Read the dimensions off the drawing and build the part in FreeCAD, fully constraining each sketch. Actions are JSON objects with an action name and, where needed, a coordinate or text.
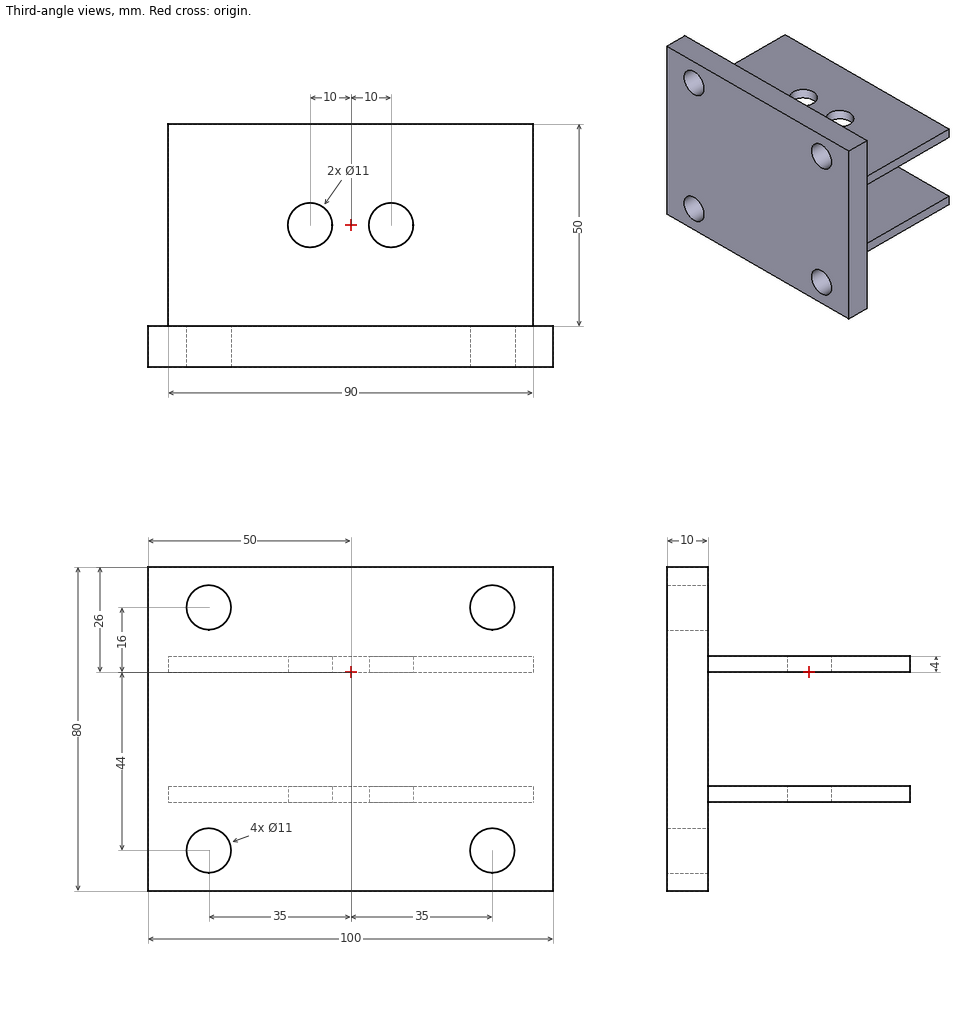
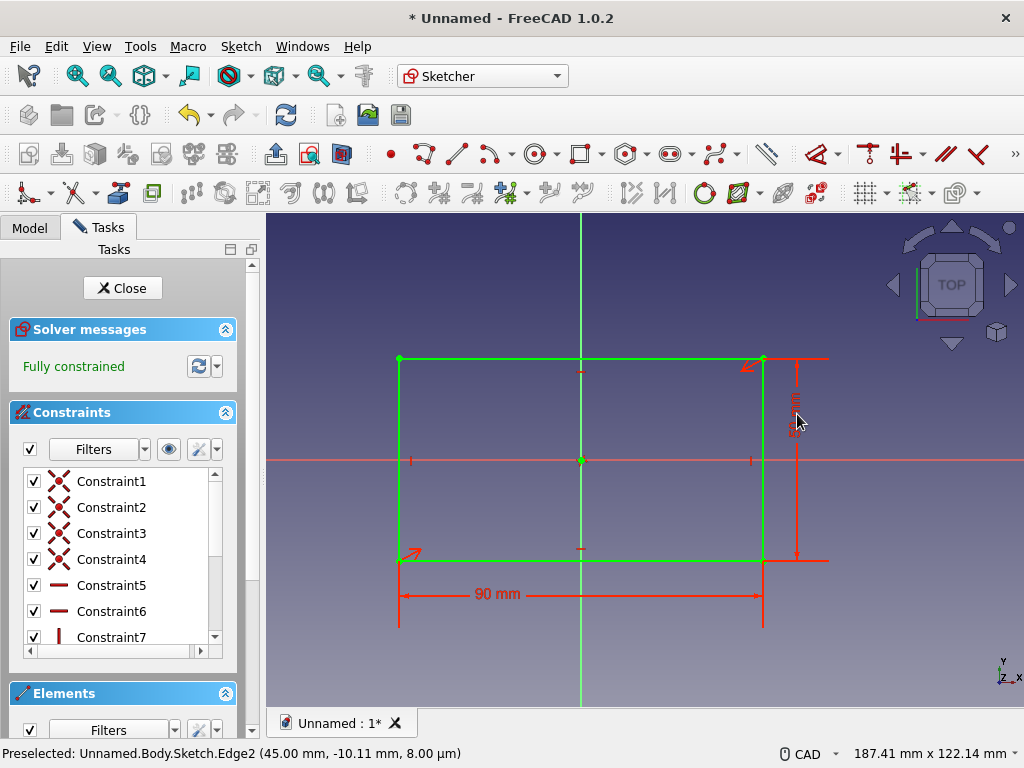
{"action": "left_click", "coordinate": [123, 288]}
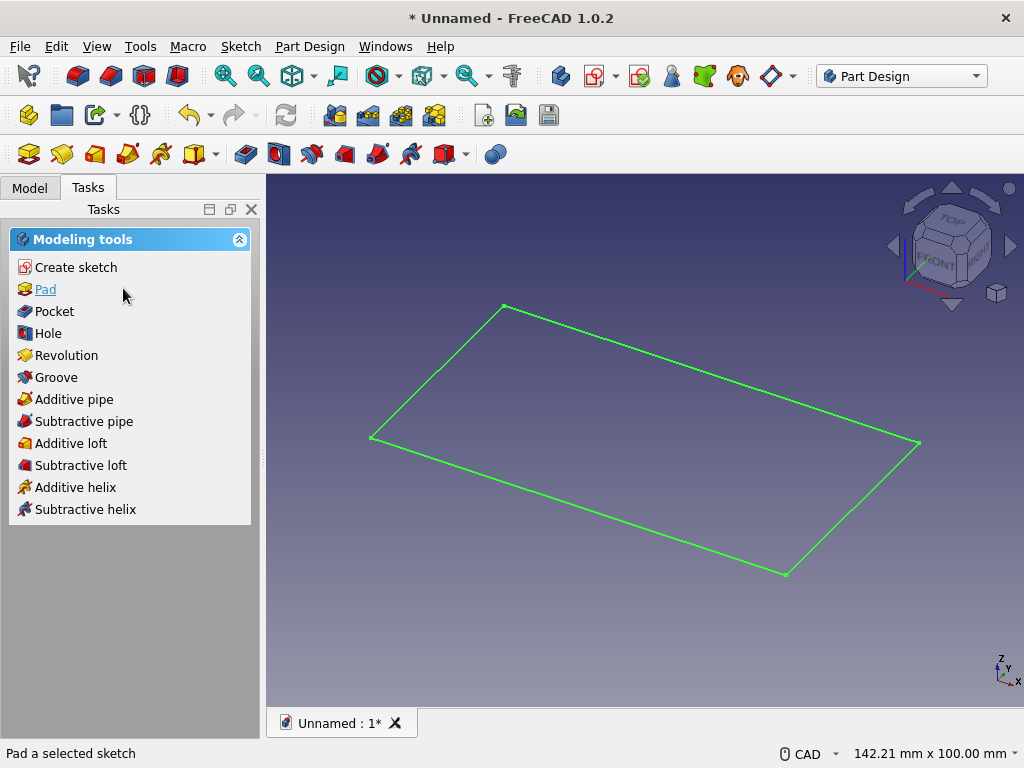
{"action": "left_click", "coordinate": [29, 154]}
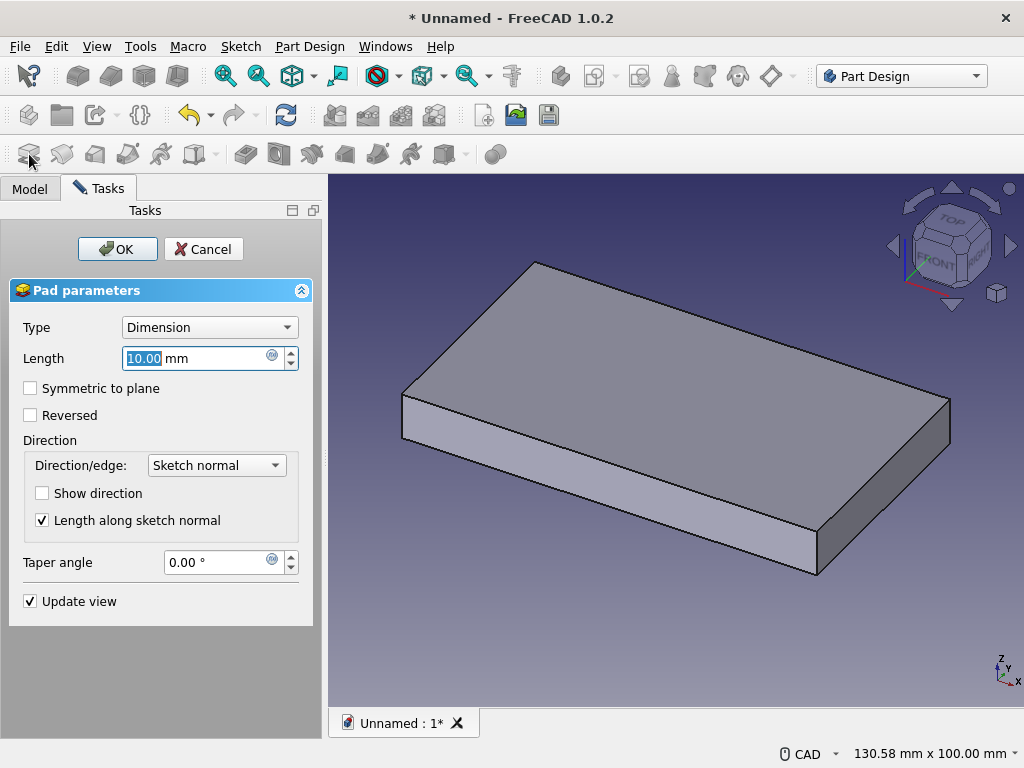
{"action": "type", "text": "4"}
{"action": "key", "text": "Tab"}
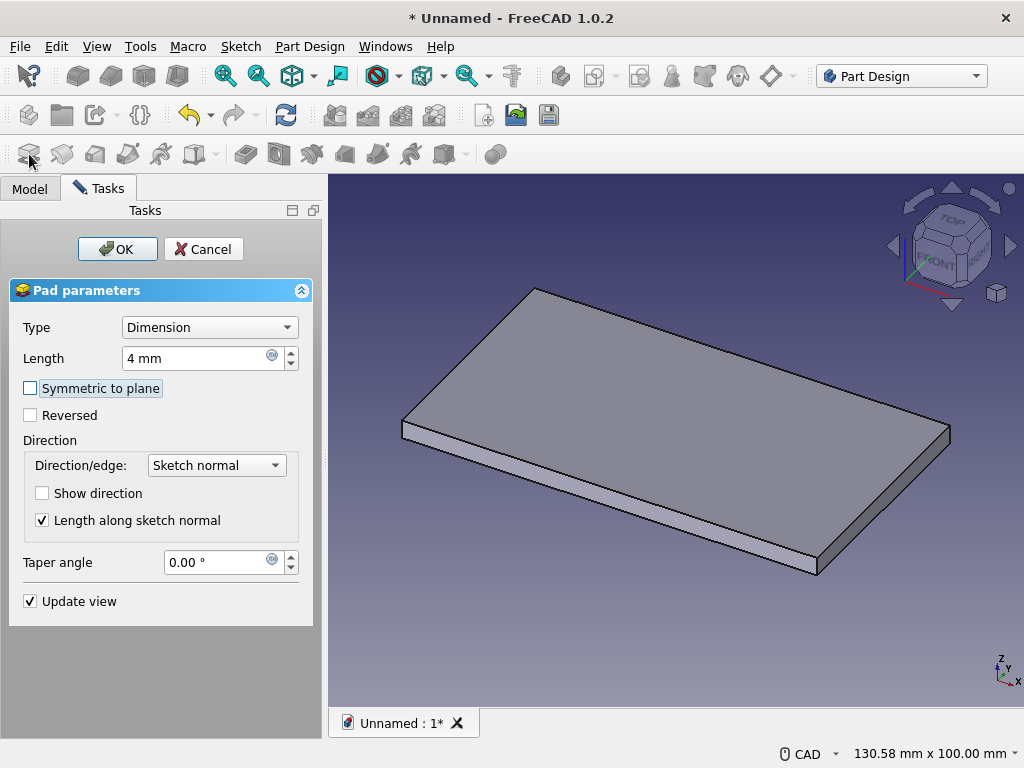
{"action": "left_click", "coordinate": [118, 249]}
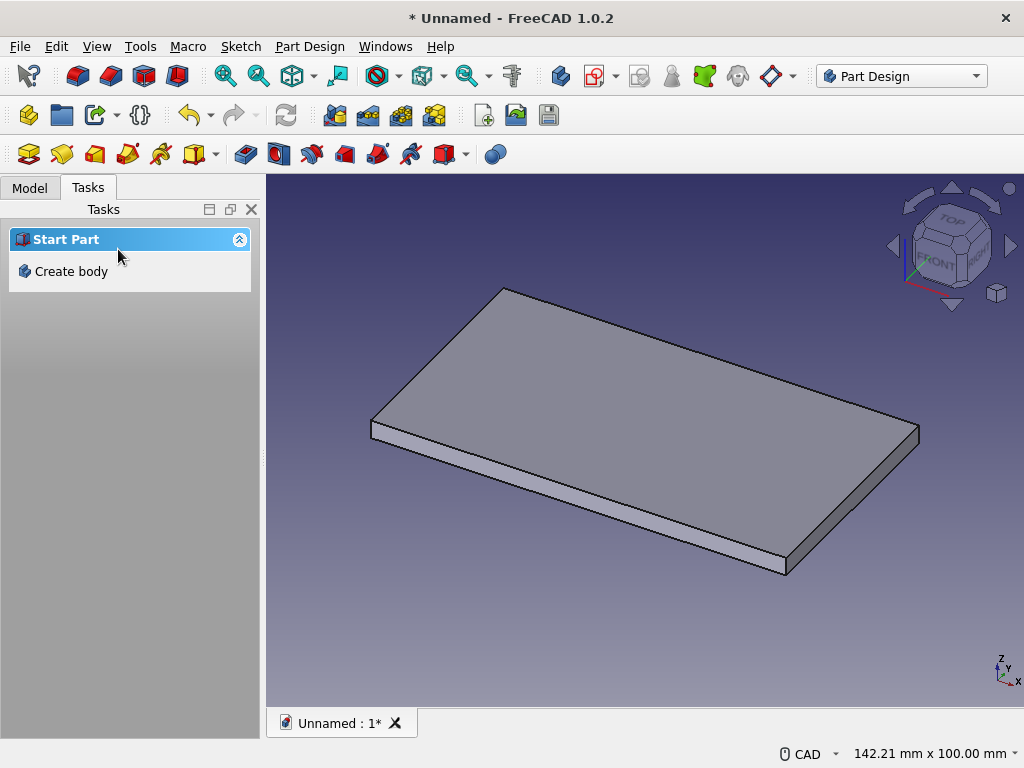
{"action": "left_click", "coordinate": [704, 442]}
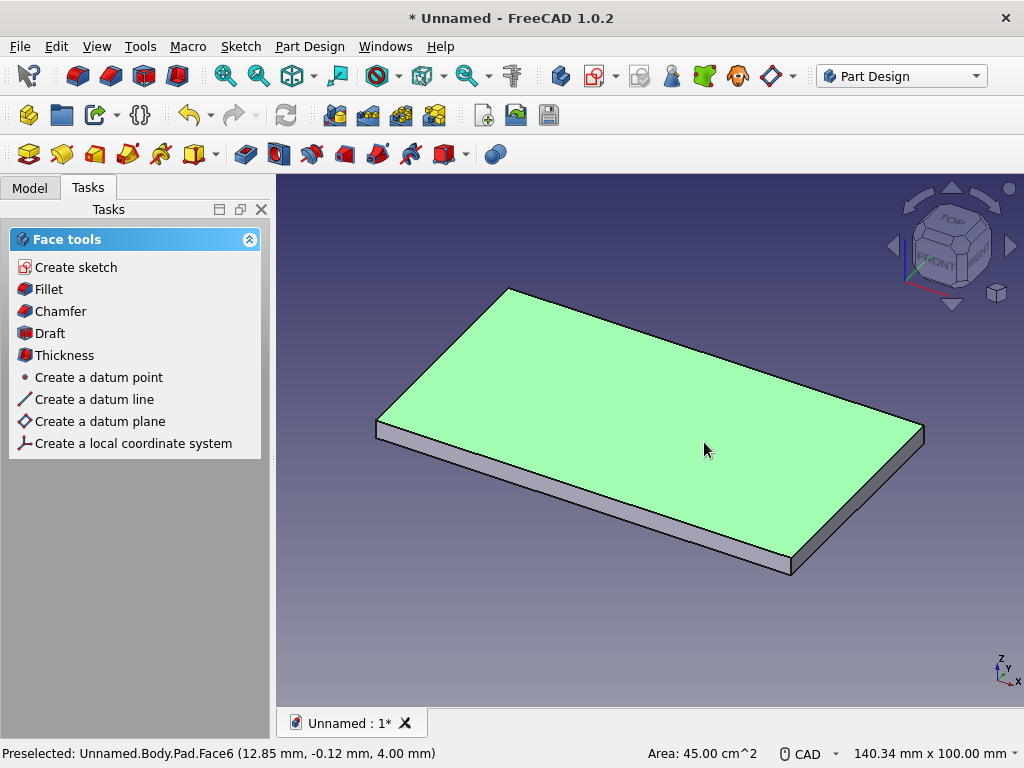
{"action": "left_click", "coordinate": [594, 76]}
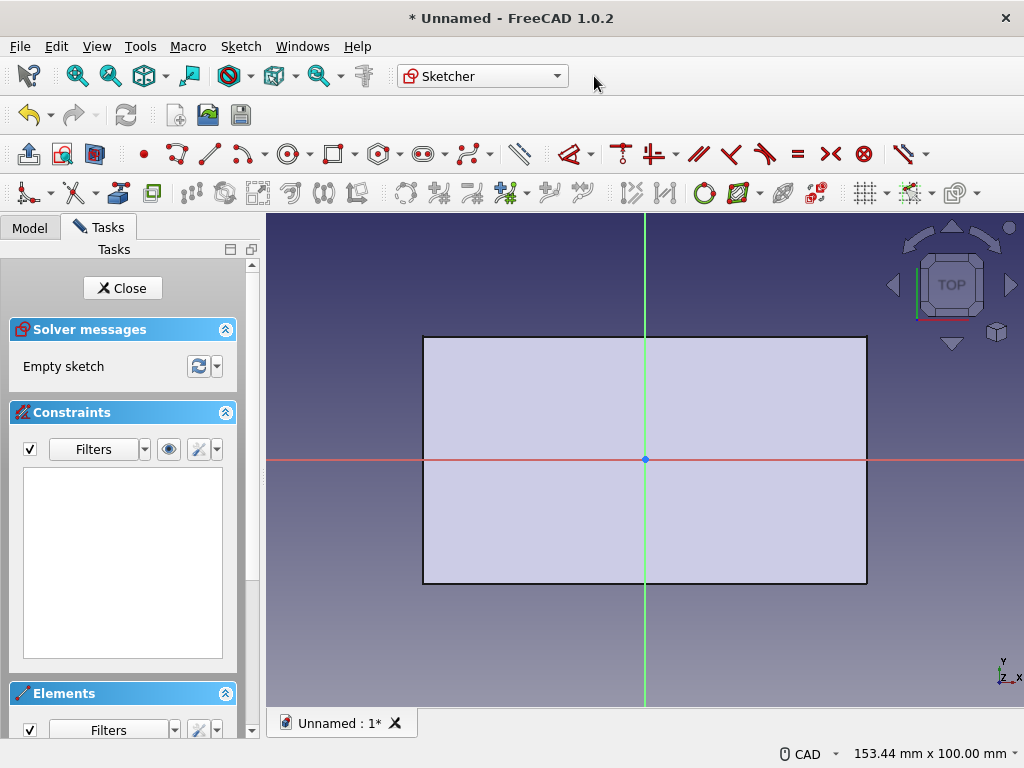
{"action": "scroll", "coordinate": [685, 460], "scroll_direction": "up", "scroll_amount": 5}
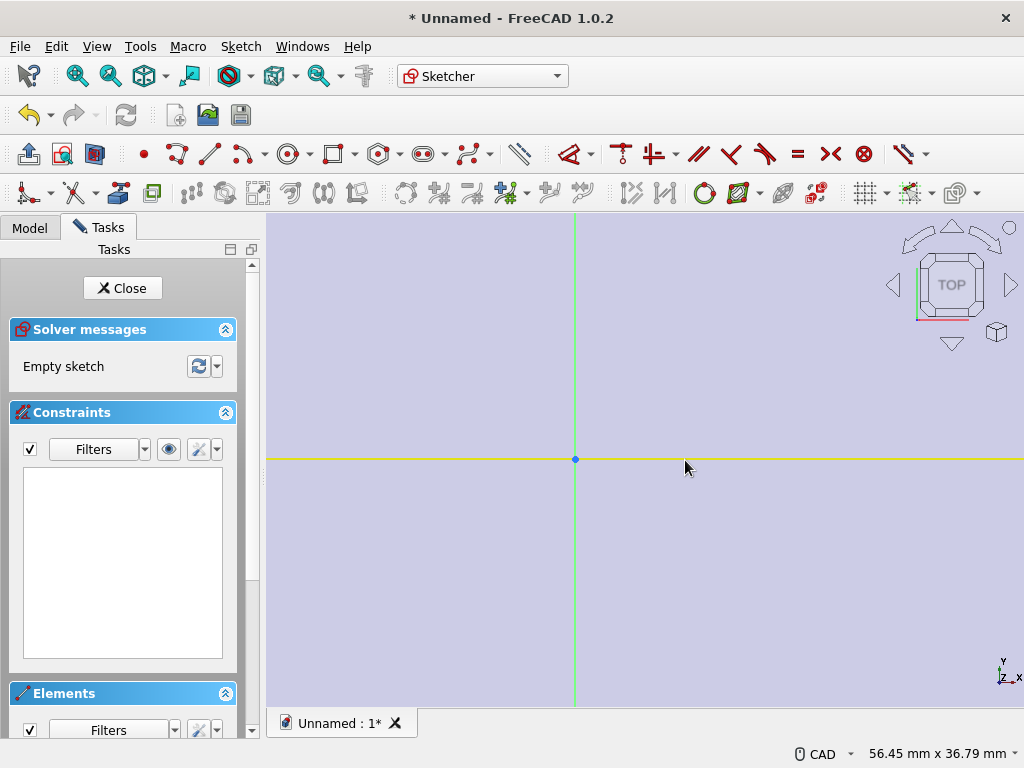
{"action": "key", "text": "g c"}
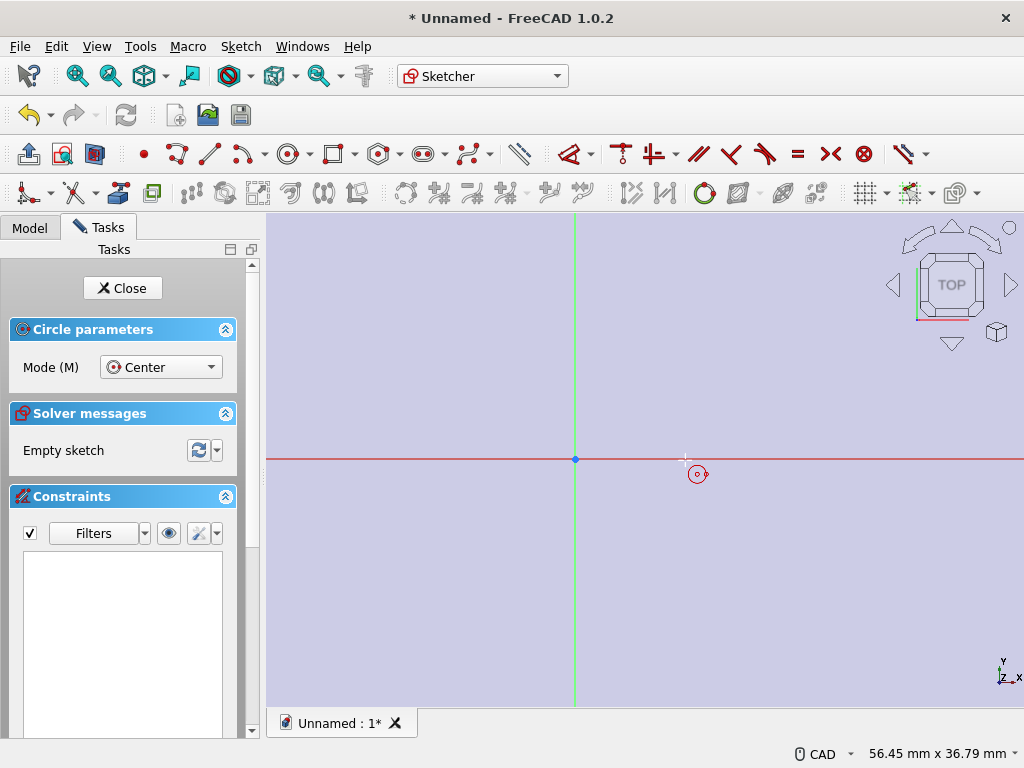
{"action": "left_click", "coordinate": [441, 459]}
{"action": "left_click", "coordinate": [493, 407]}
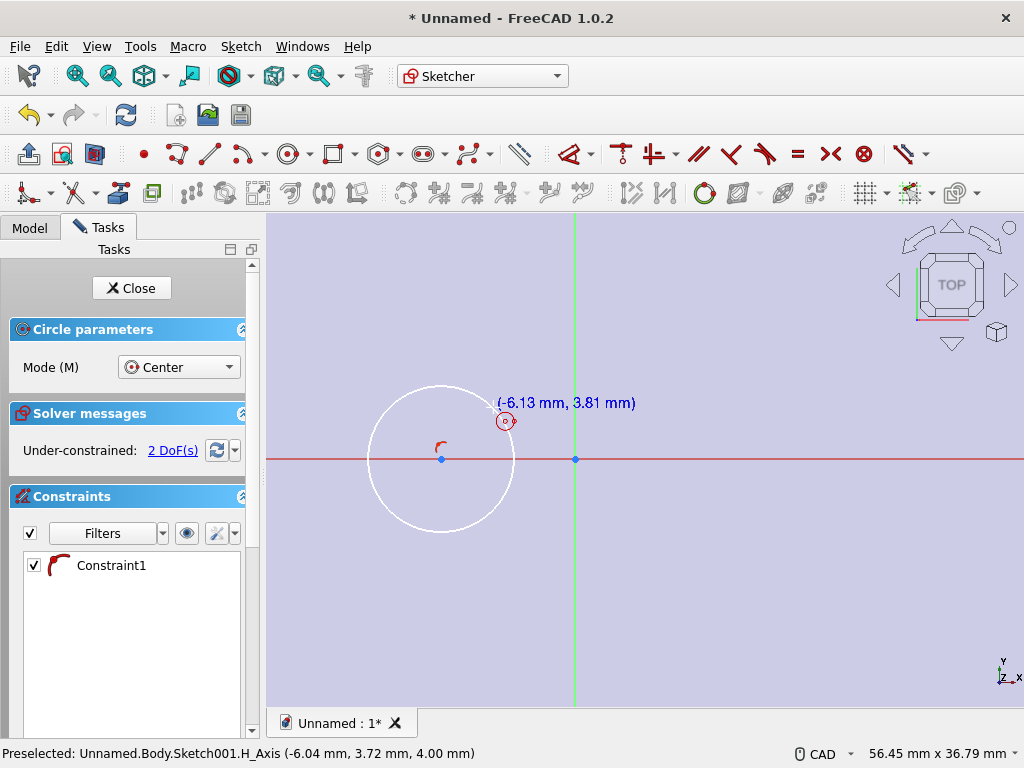
{"action": "left_click", "coordinate": [710, 459]}
{"action": "left_click", "coordinate": [762, 407]}
{"action": "key", "text": "Escape"}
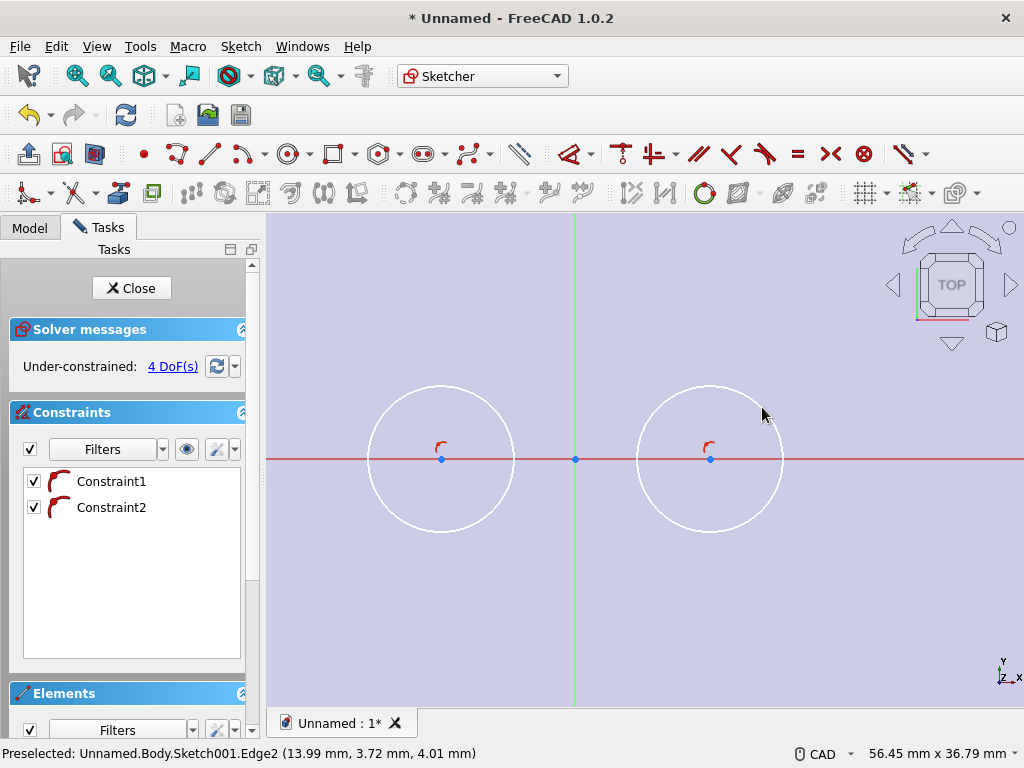
{"action": "left_click", "coordinate": [492, 407]}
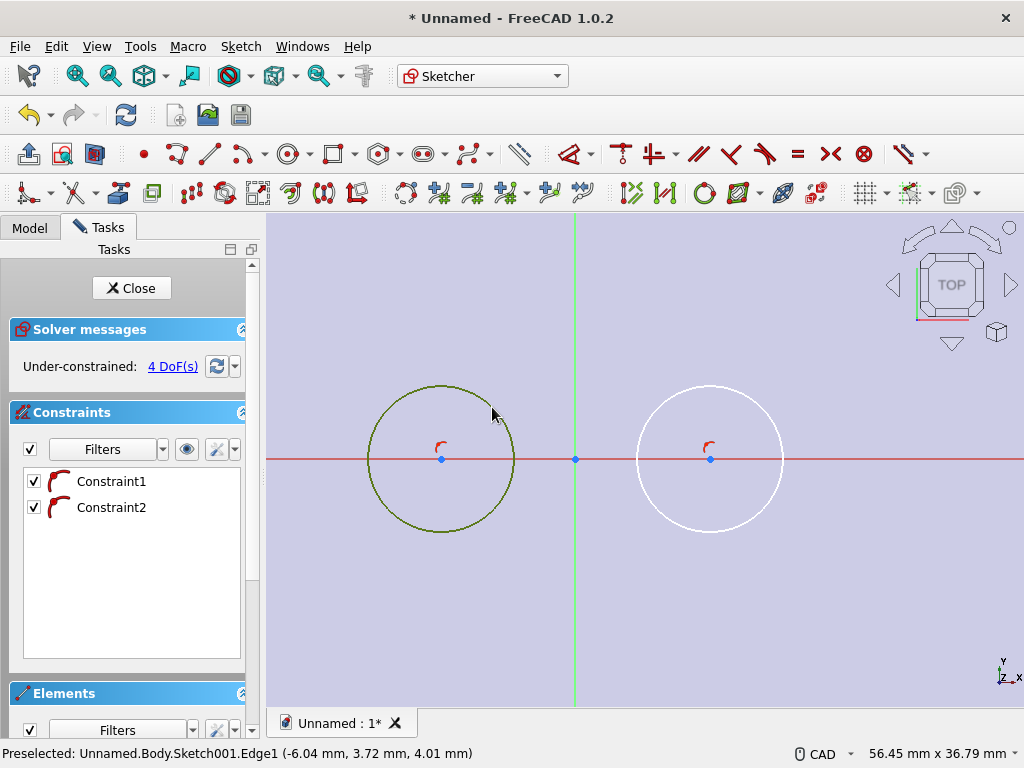
{"action": "left_click", "coordinate": [761, 407]}